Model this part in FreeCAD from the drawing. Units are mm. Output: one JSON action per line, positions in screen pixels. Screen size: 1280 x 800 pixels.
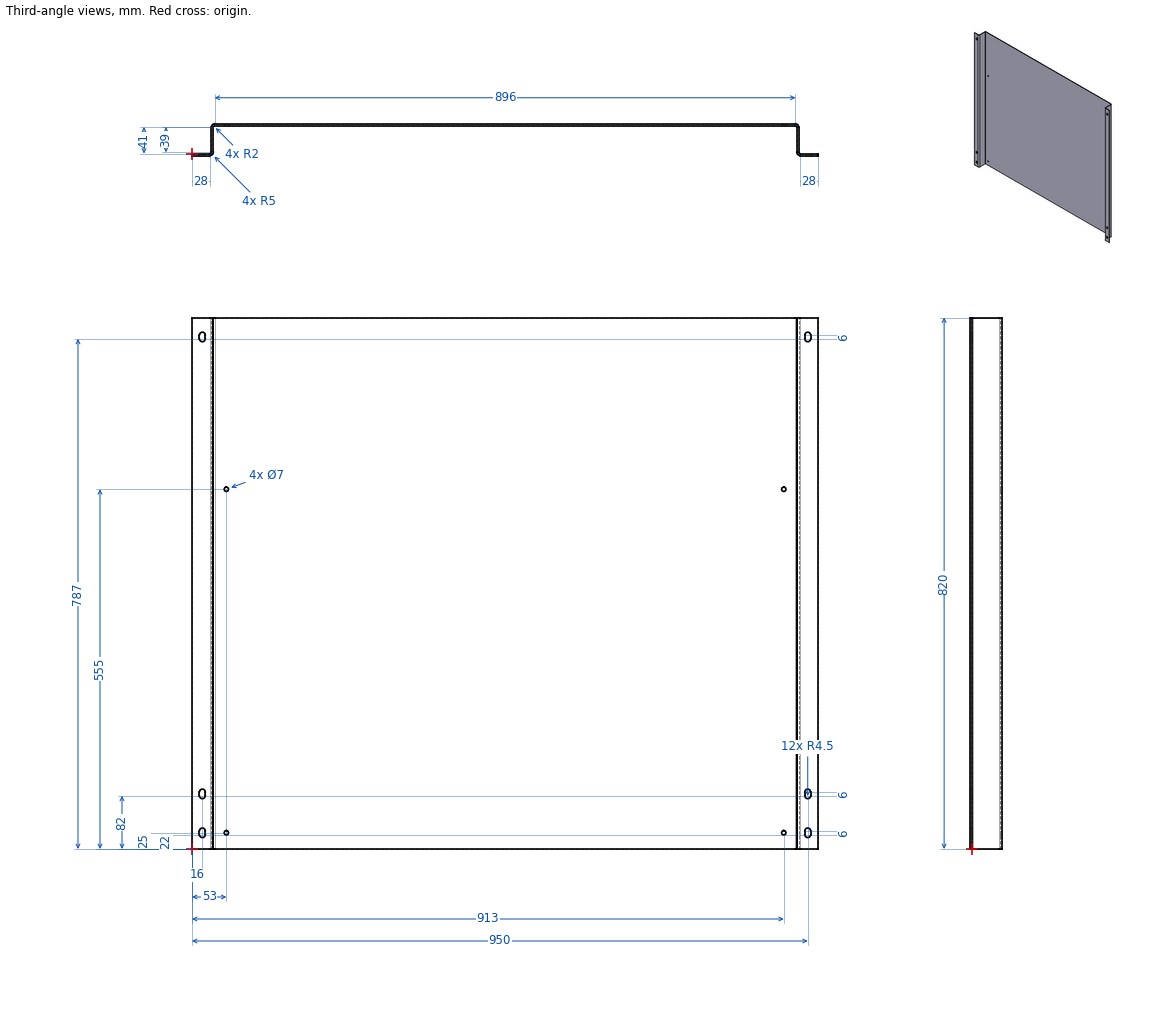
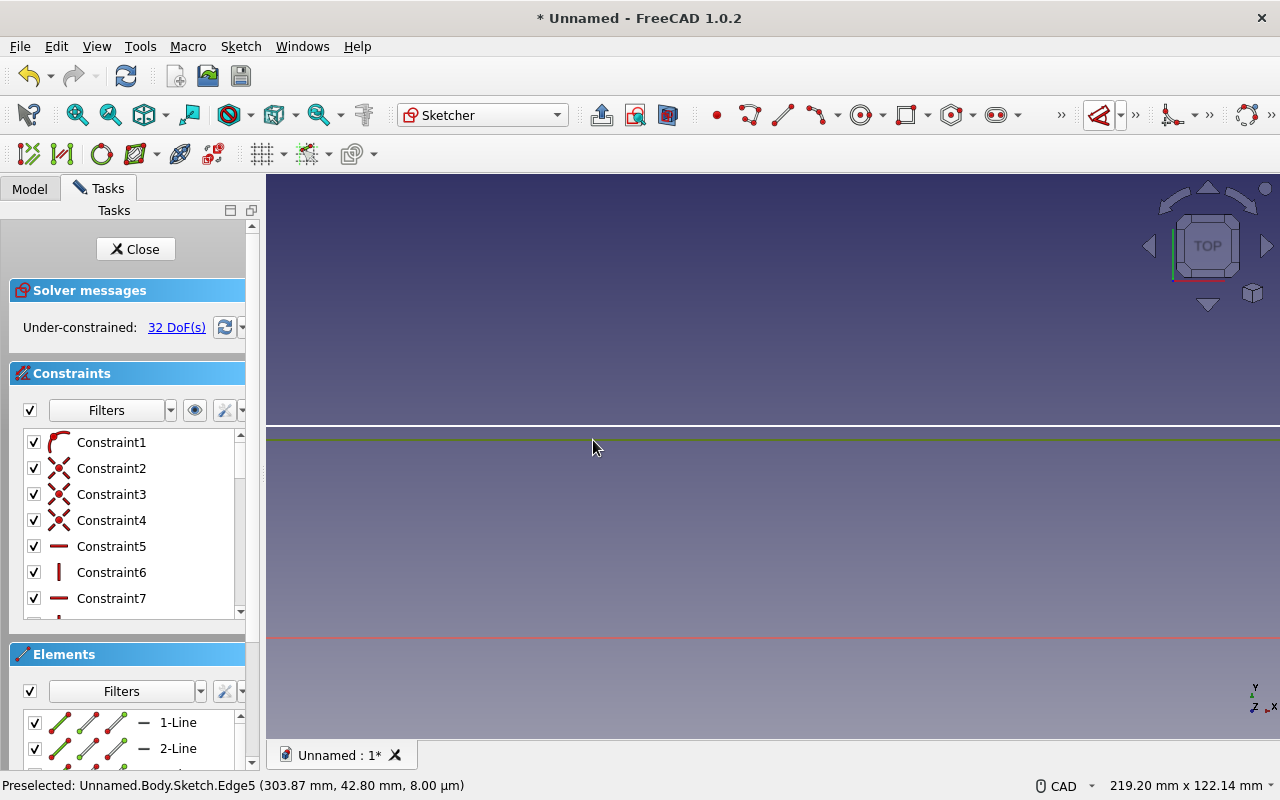
{"action": "scroll", "coordinate": [592, 444], "scroll_direction": "down", "scroll_amount": 10}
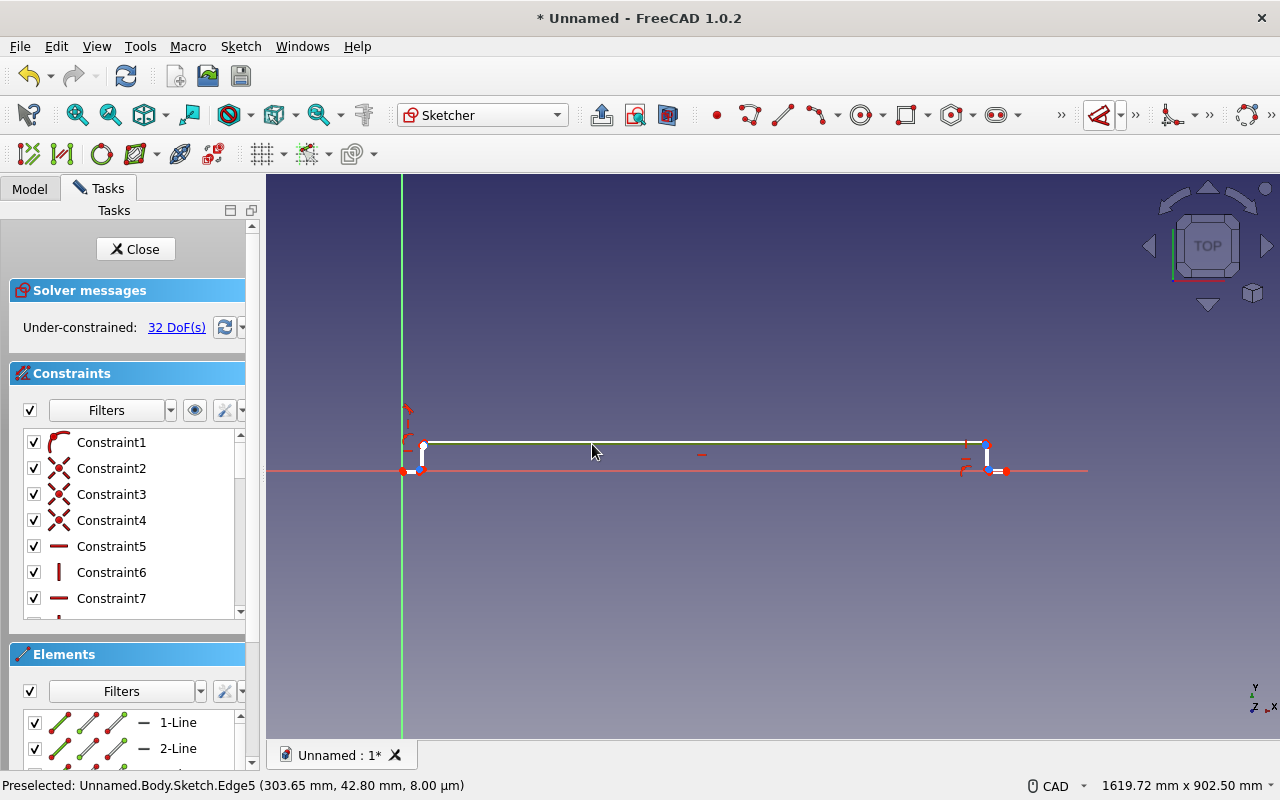
{"action": "scroll", "coordinate": [986, 444], "scroll_direction": "up", "scroll_amount": 14}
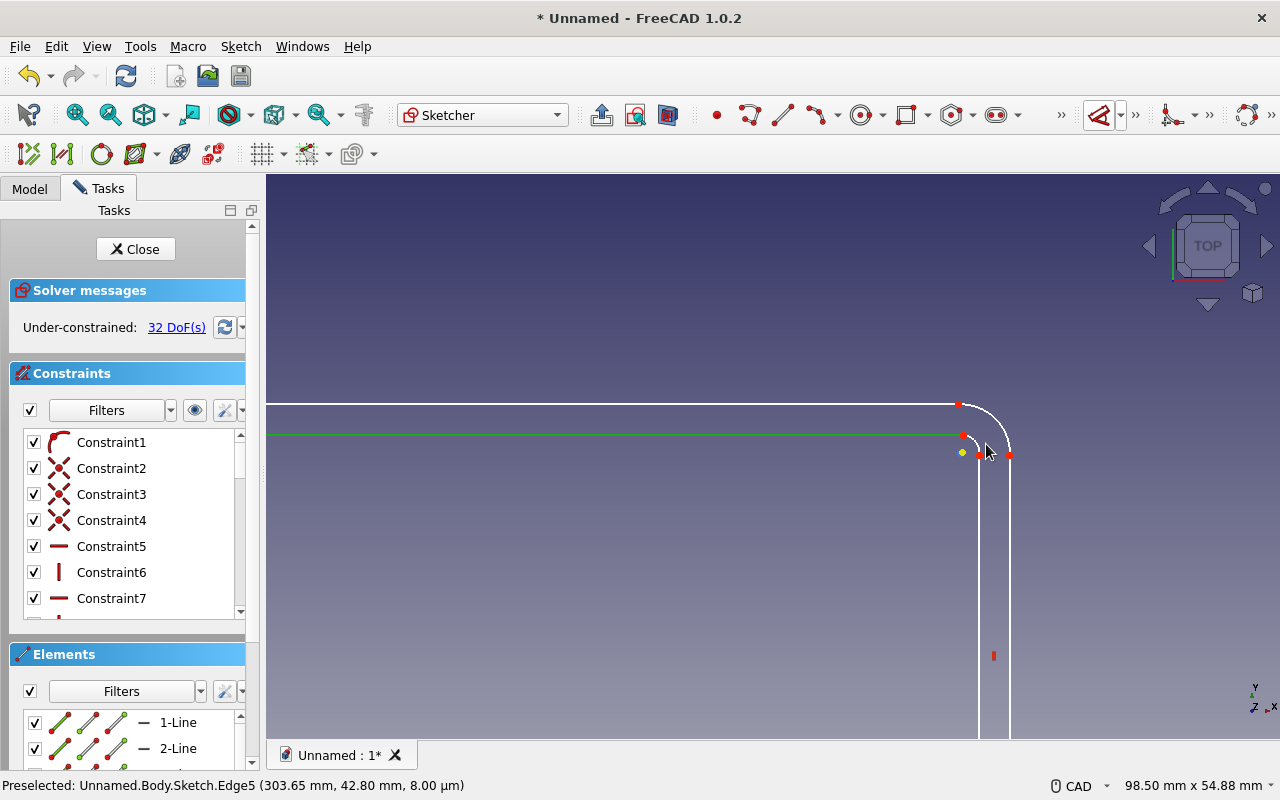
{"action": "left_click", "coordinate": [976, 442]}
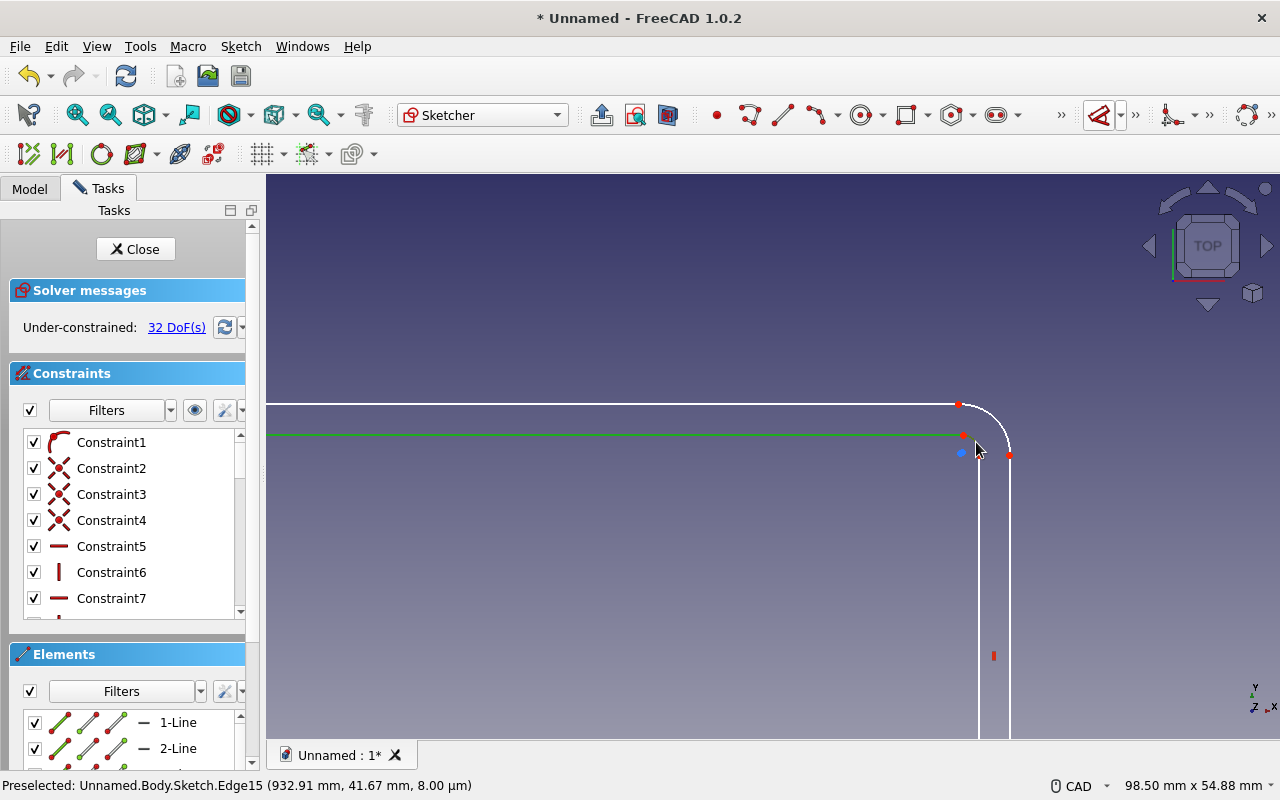
{"action": "key", "text": "t"}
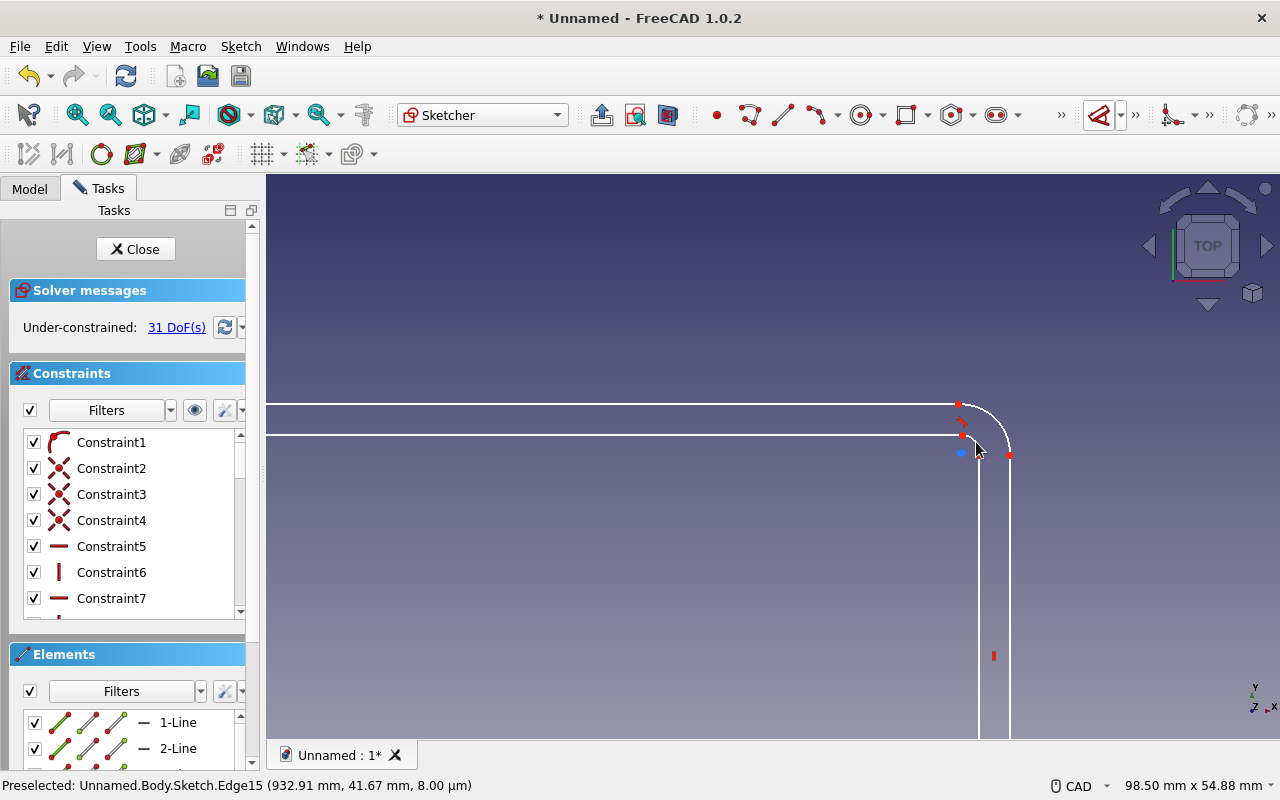
{"action": "left_click", "coordinate": [979, 576]}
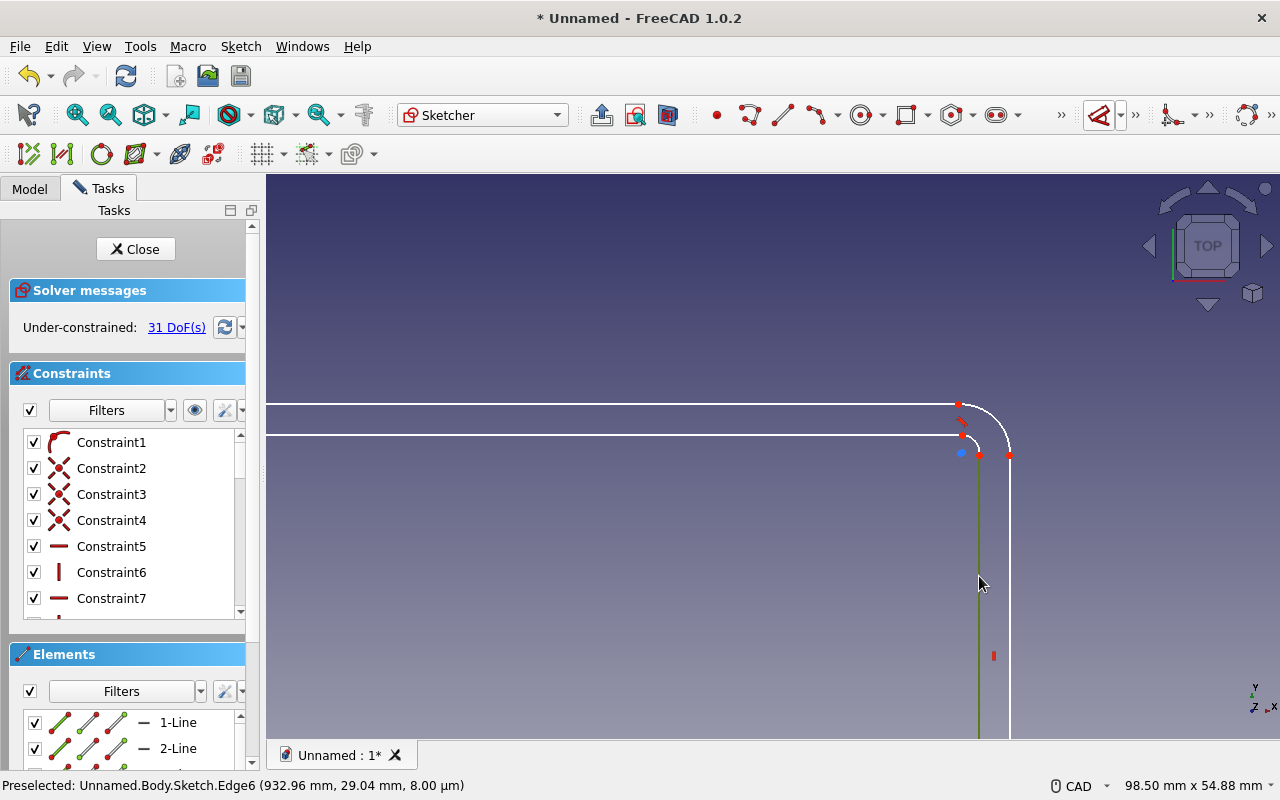
{"action": "left_click", "coordinate": [975, 441]}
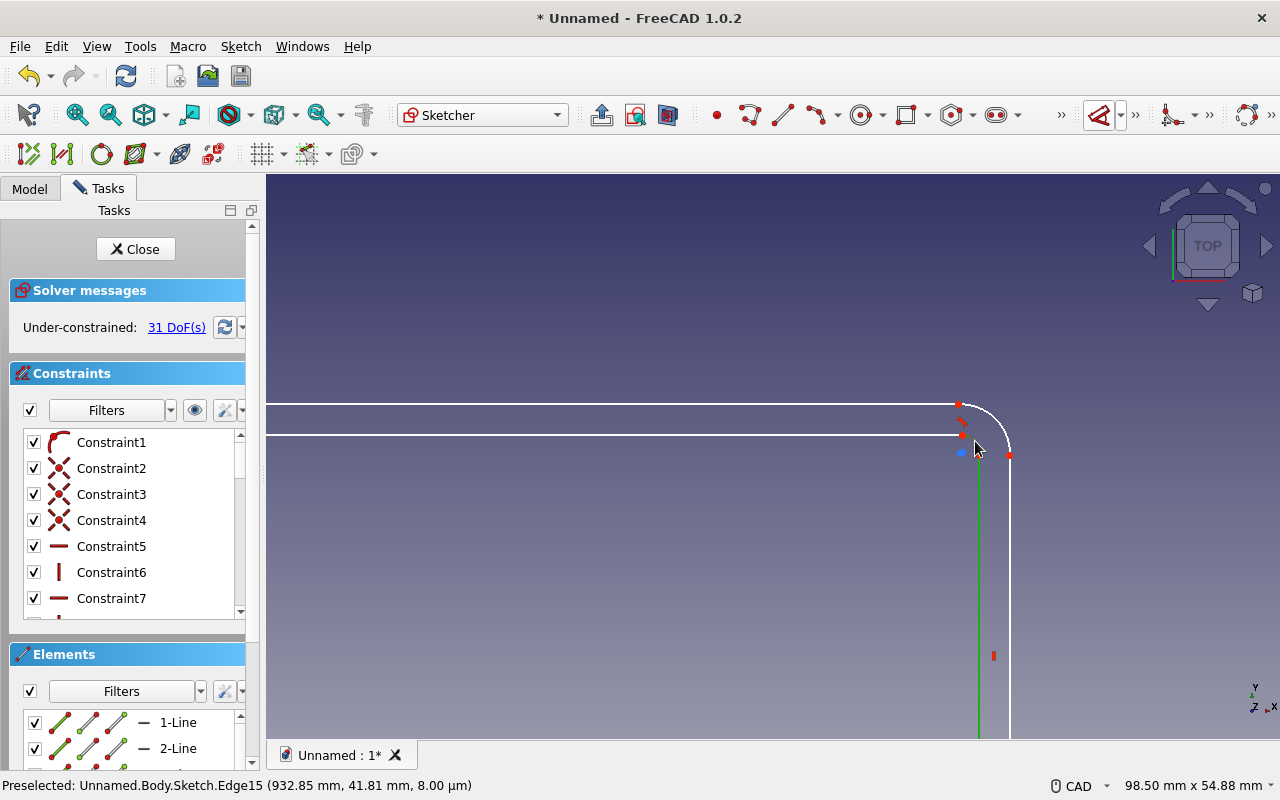
{"action": "key", "text": "t"}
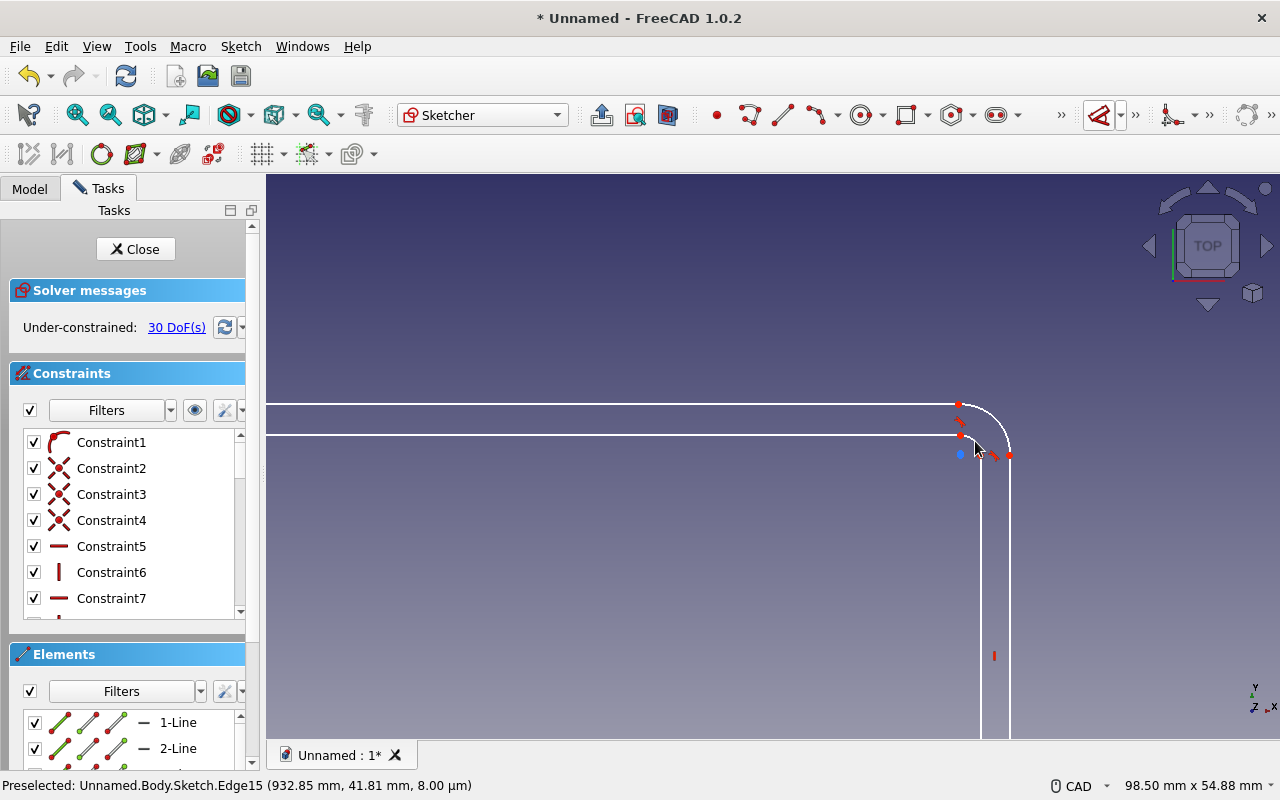
{"action": "left_click", "coordinate": [981, 576]}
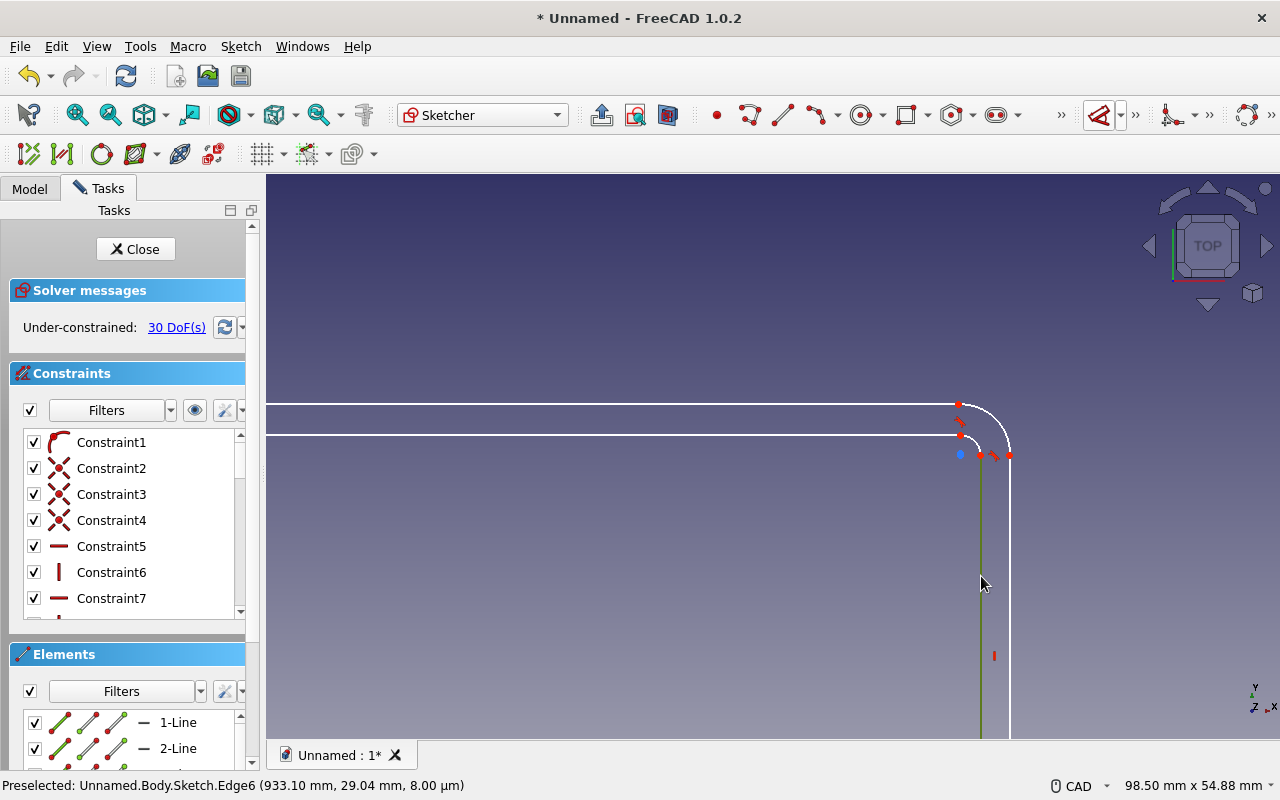
{"action": "scroll", "coordinate": [987, 444], "scroll_direction": "down", "scroll_amount": 14}